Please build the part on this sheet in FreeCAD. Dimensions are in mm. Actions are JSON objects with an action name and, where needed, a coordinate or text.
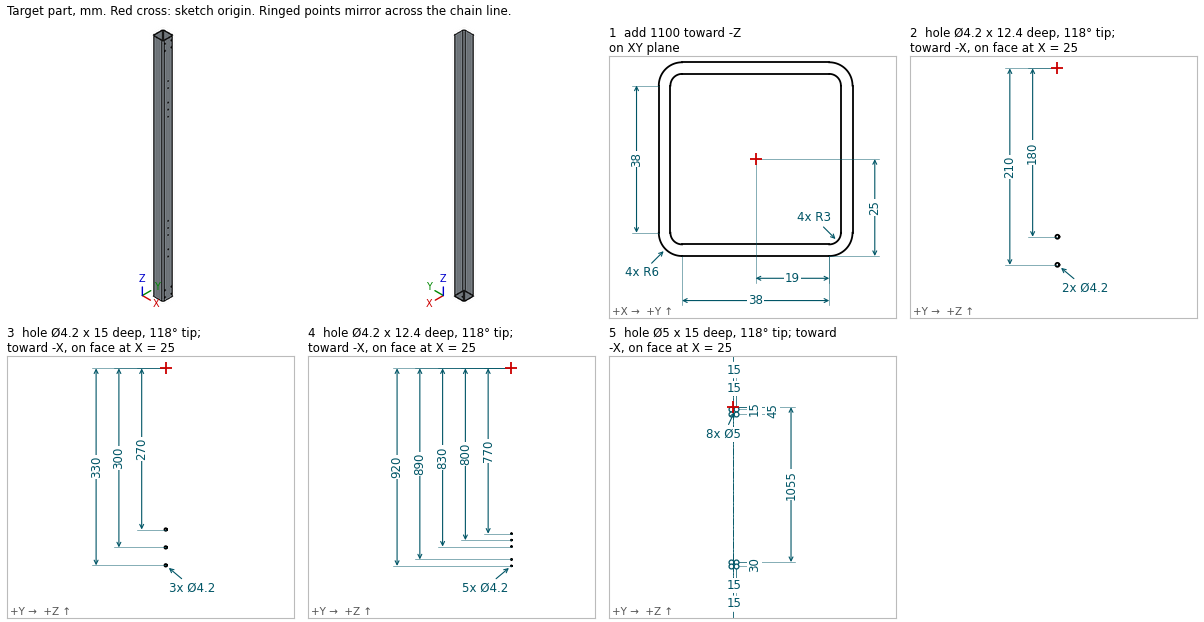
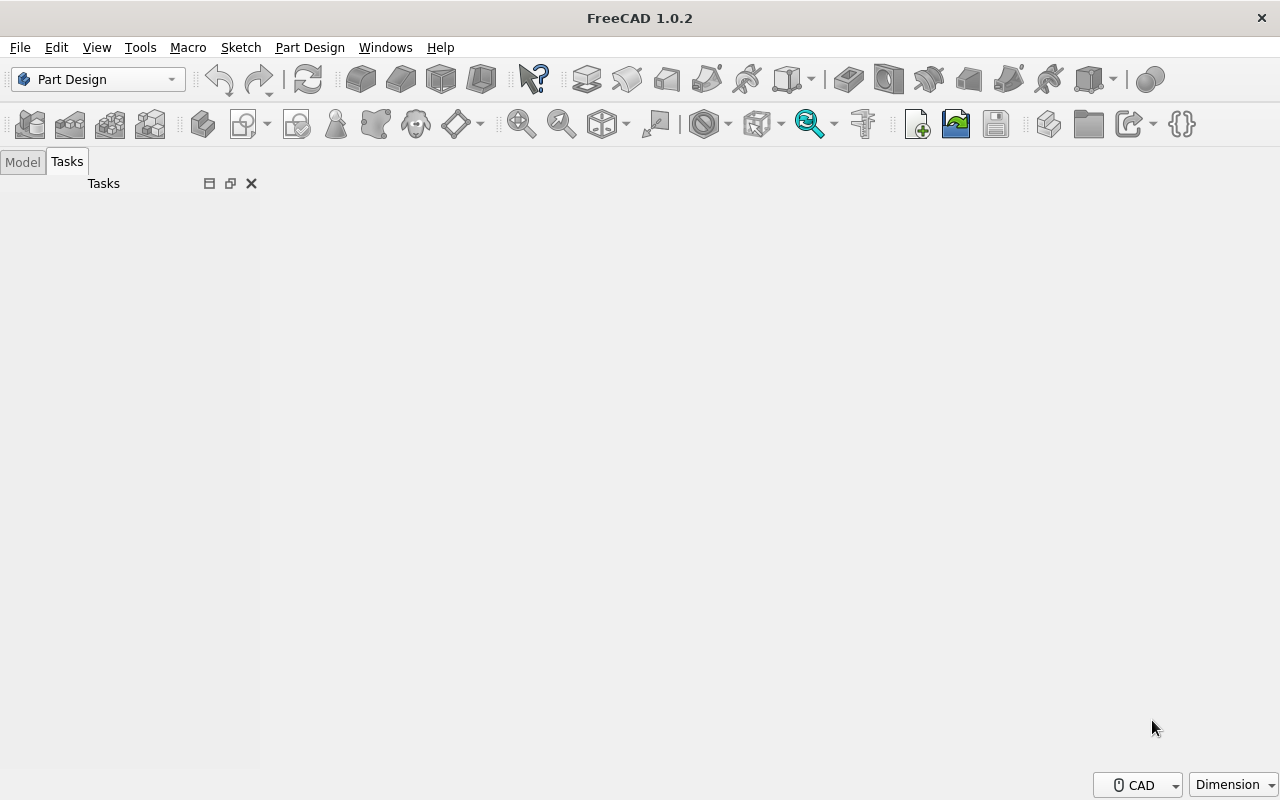
{"action": "left_click", "coordinate": [916, 124]}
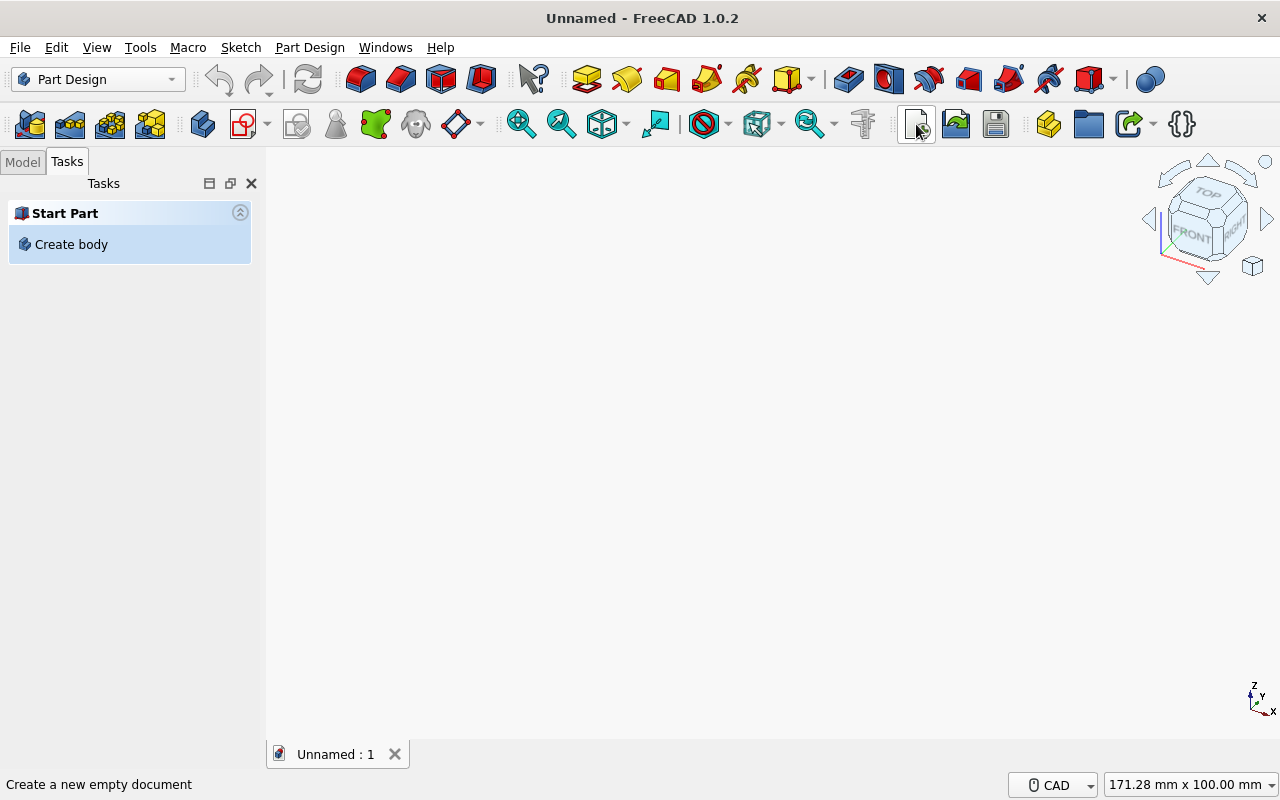
{"action": "left_click", "coordinate": [244, 124]}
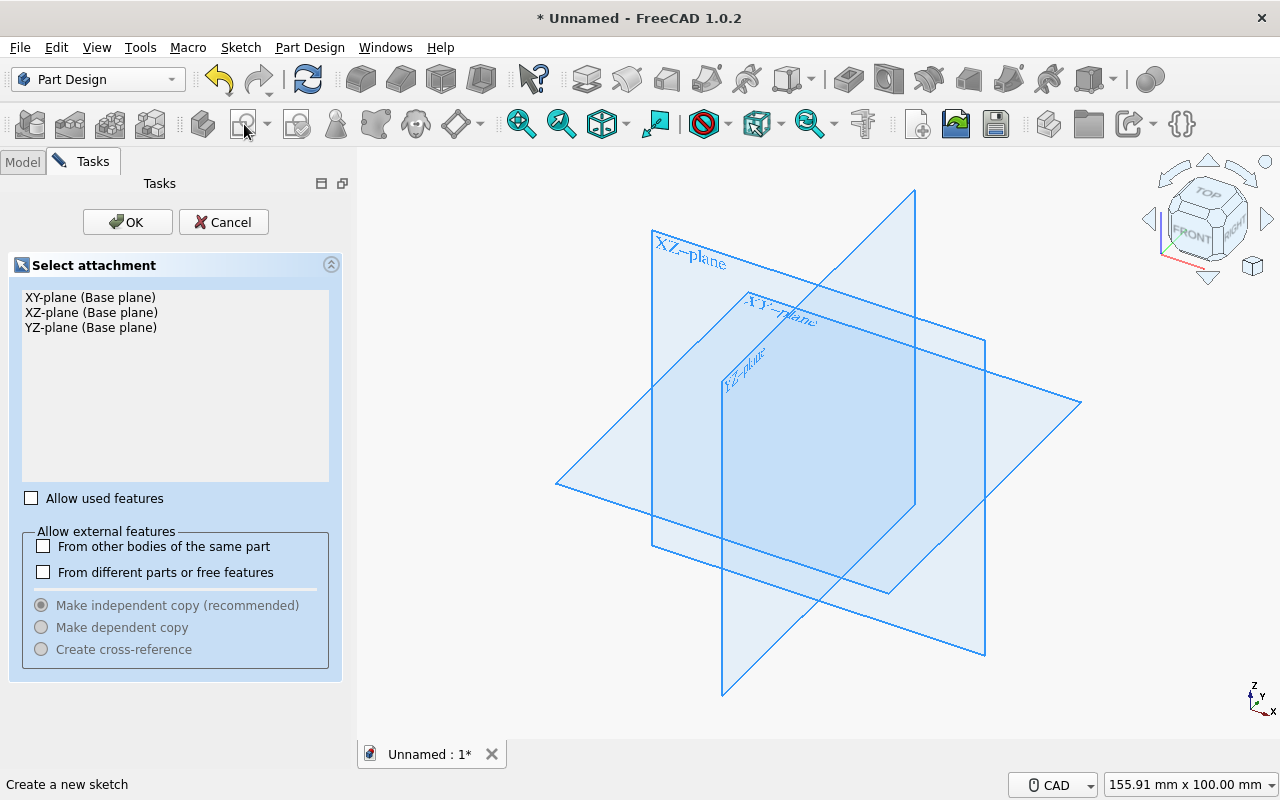
{"action": "left_click", "coordinate": [82, 298]}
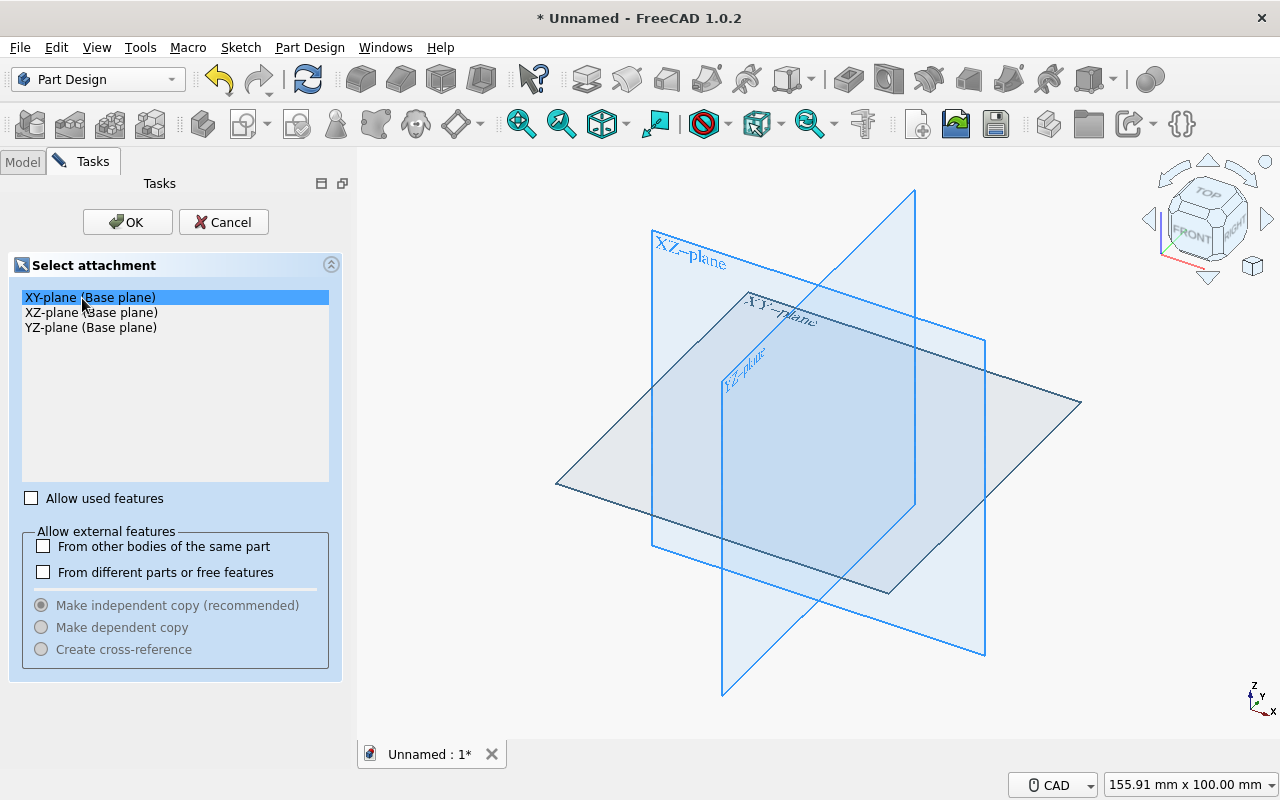
{"action": "left_click", "coordinate": [128, 222]}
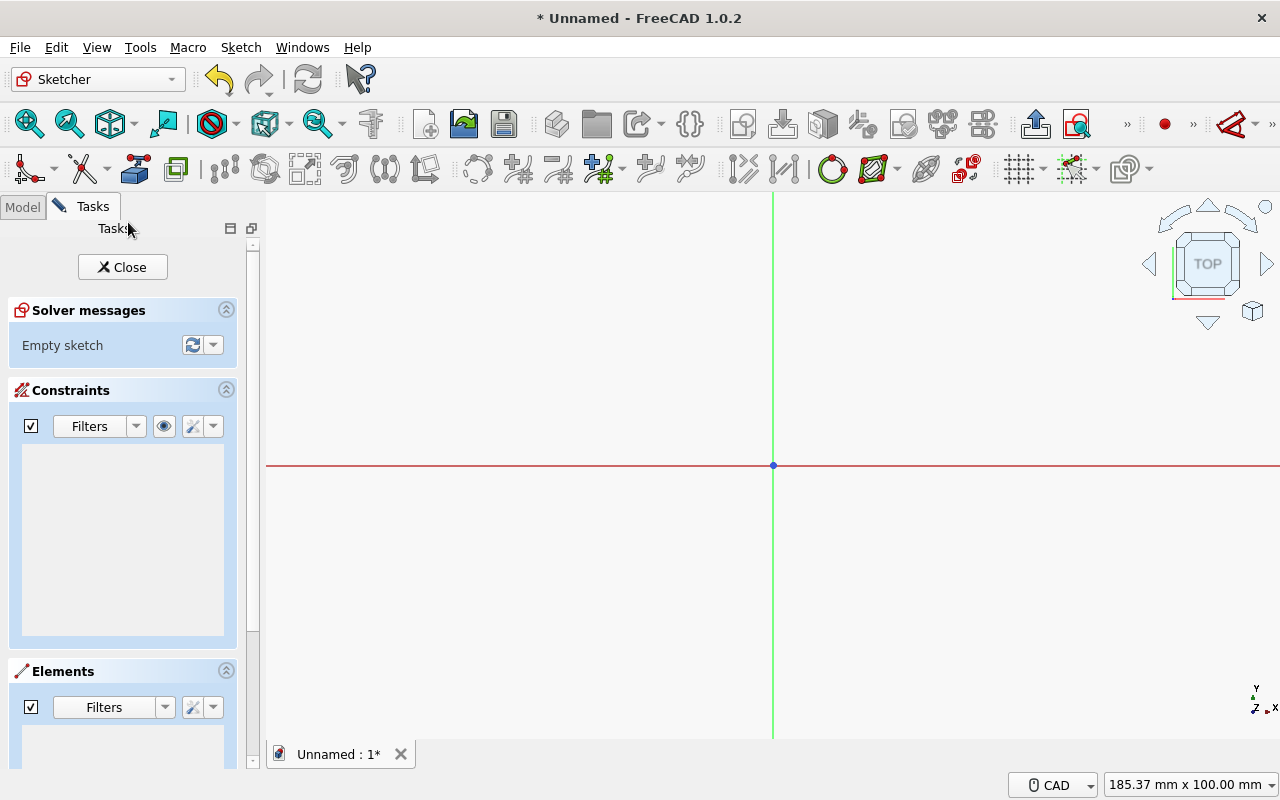
{"action": "key", "text": "g l"}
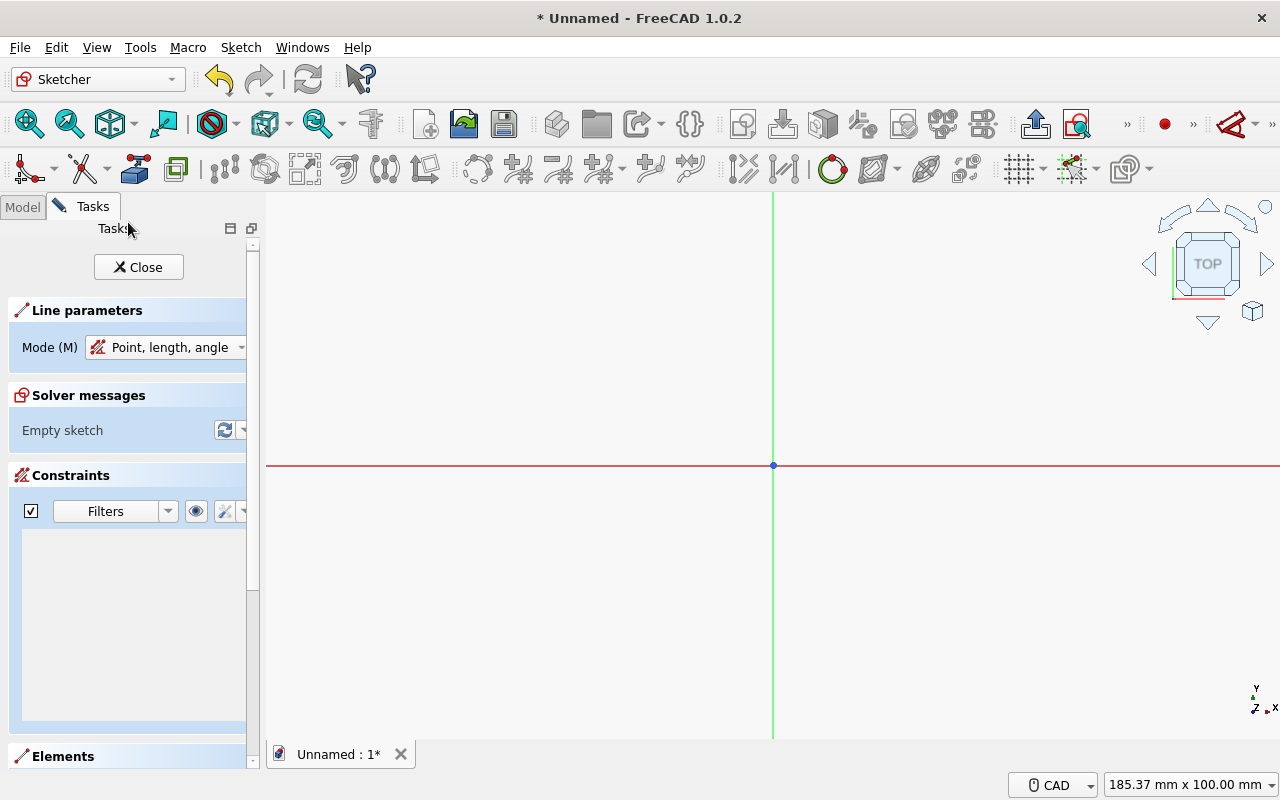
{"action": "left_click", "coordinate": [877, 602]}
{"action": "left_click", "coordinate": [669, 602]}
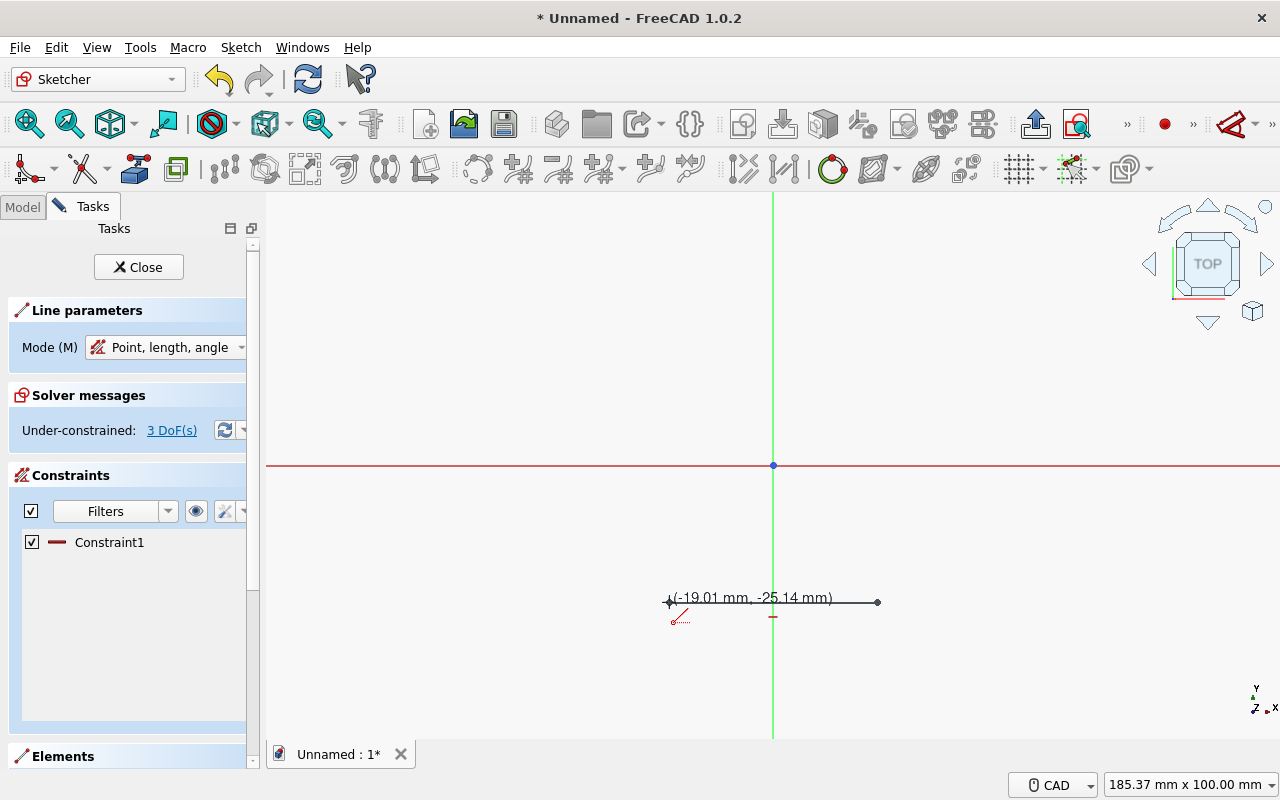
{"action": "left_click", "coordinate": [636, 569]}
{"action": "left_click", "coordinate": [636, 362]}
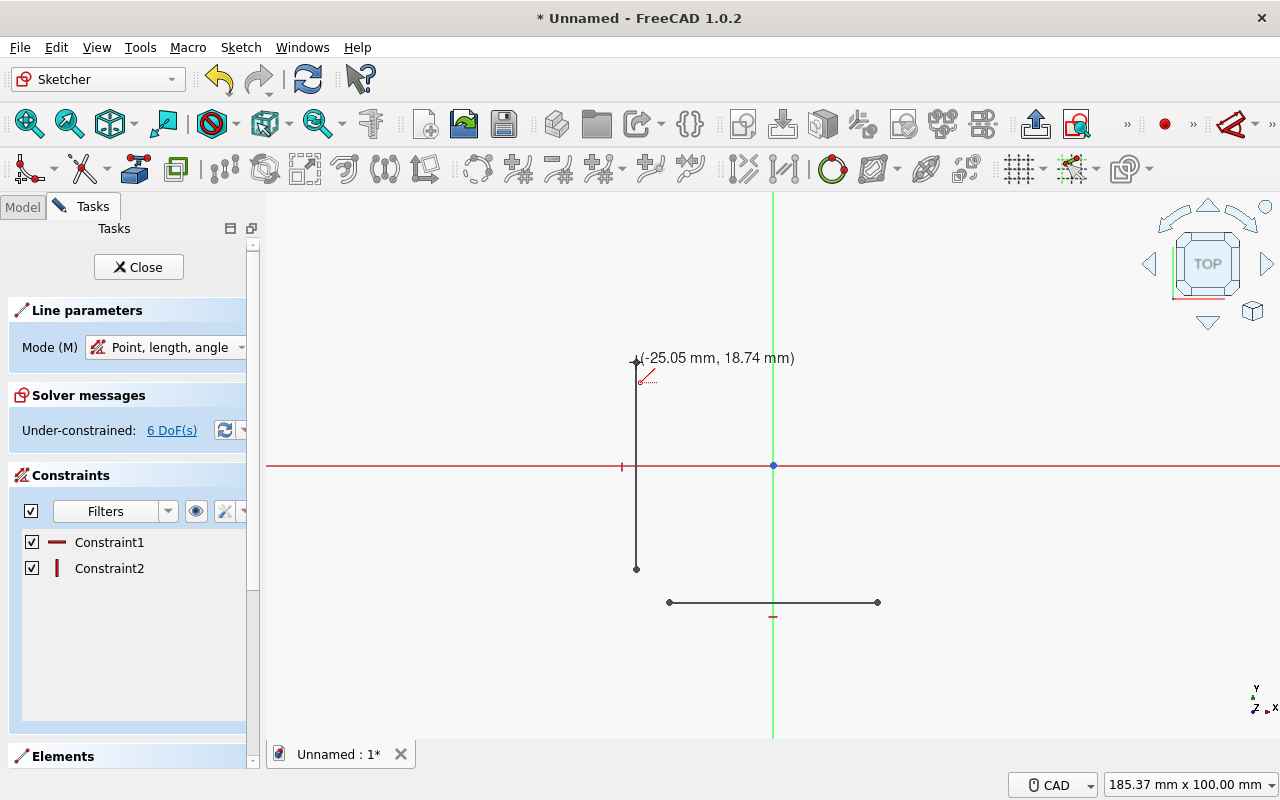
{"action": "left_click", "coordinate": [669, 329]}
{"action": "left_click", "coordinate": [877, 329]}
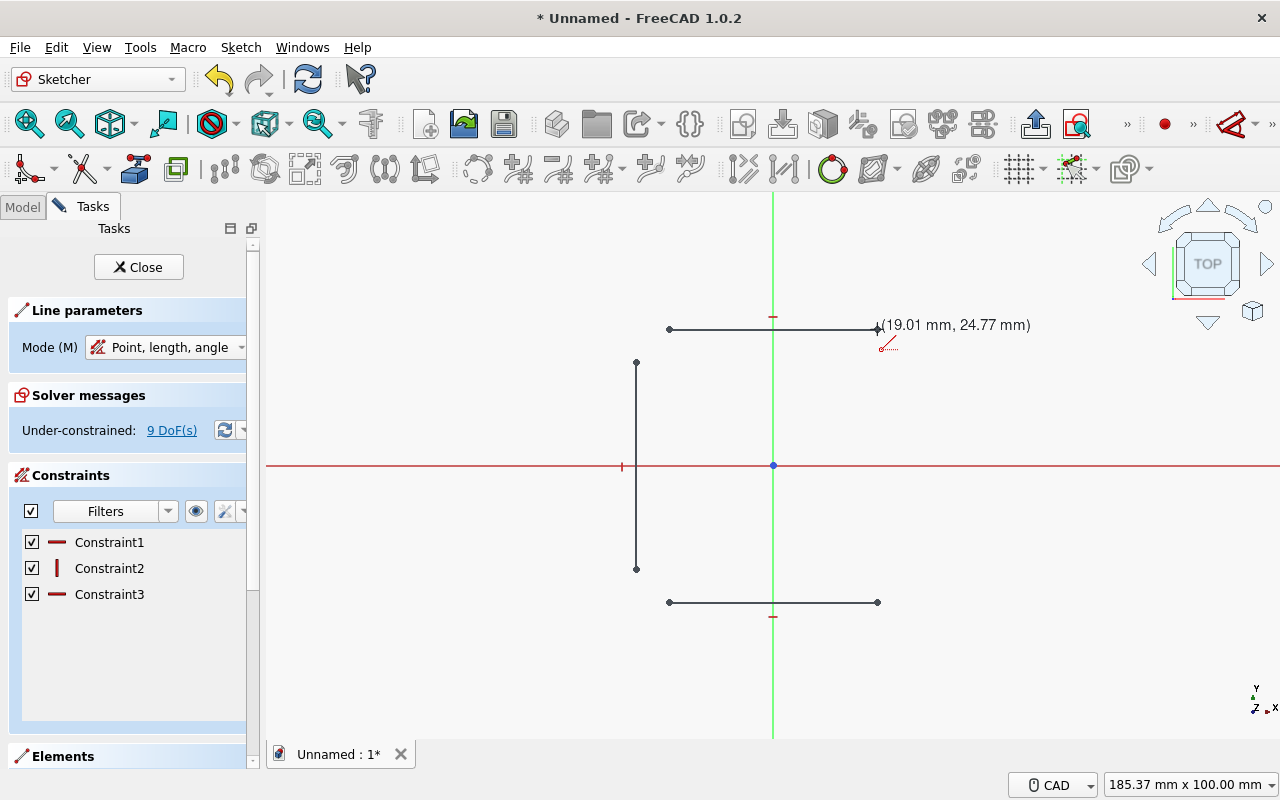
{"action": "left_click", "coordinate": [910, 362]}
{"action": "left_click", "coordinate": [910, 569]}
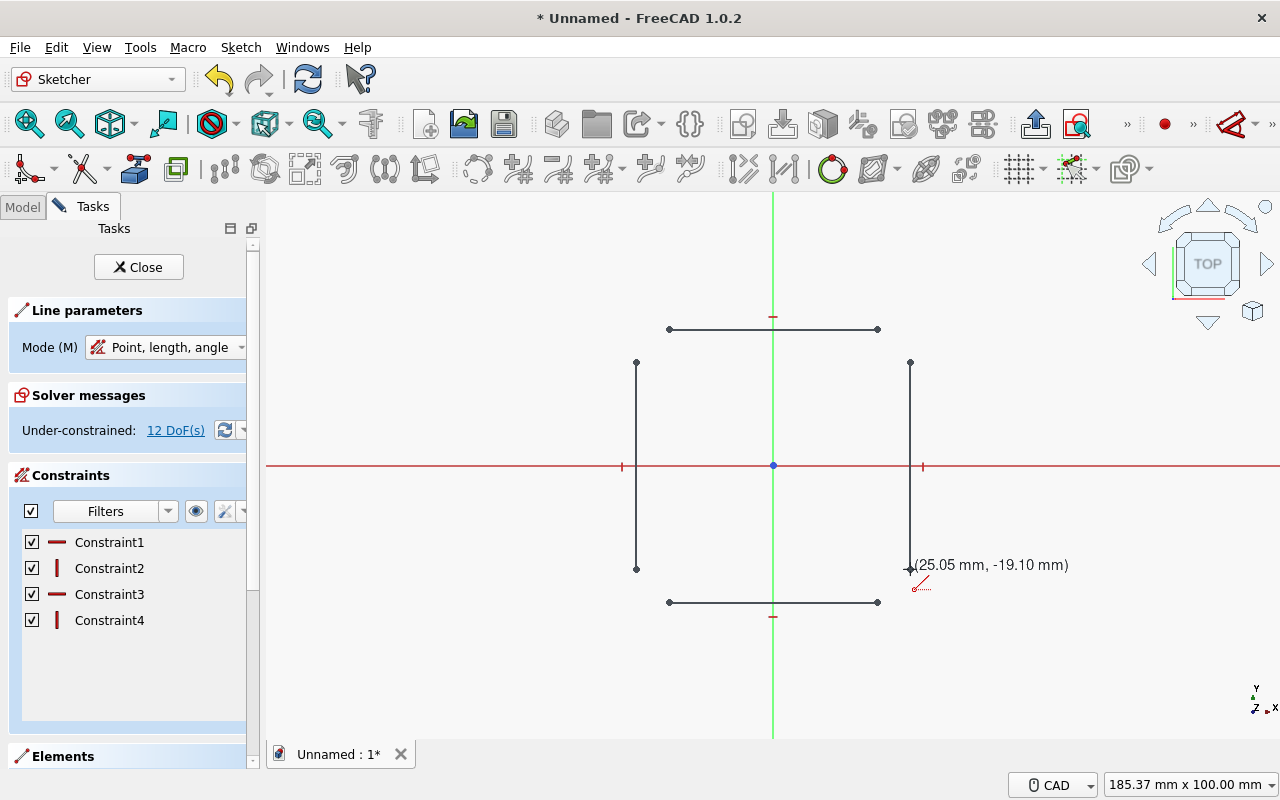
{"action": "key", "text": "g 3 a"}